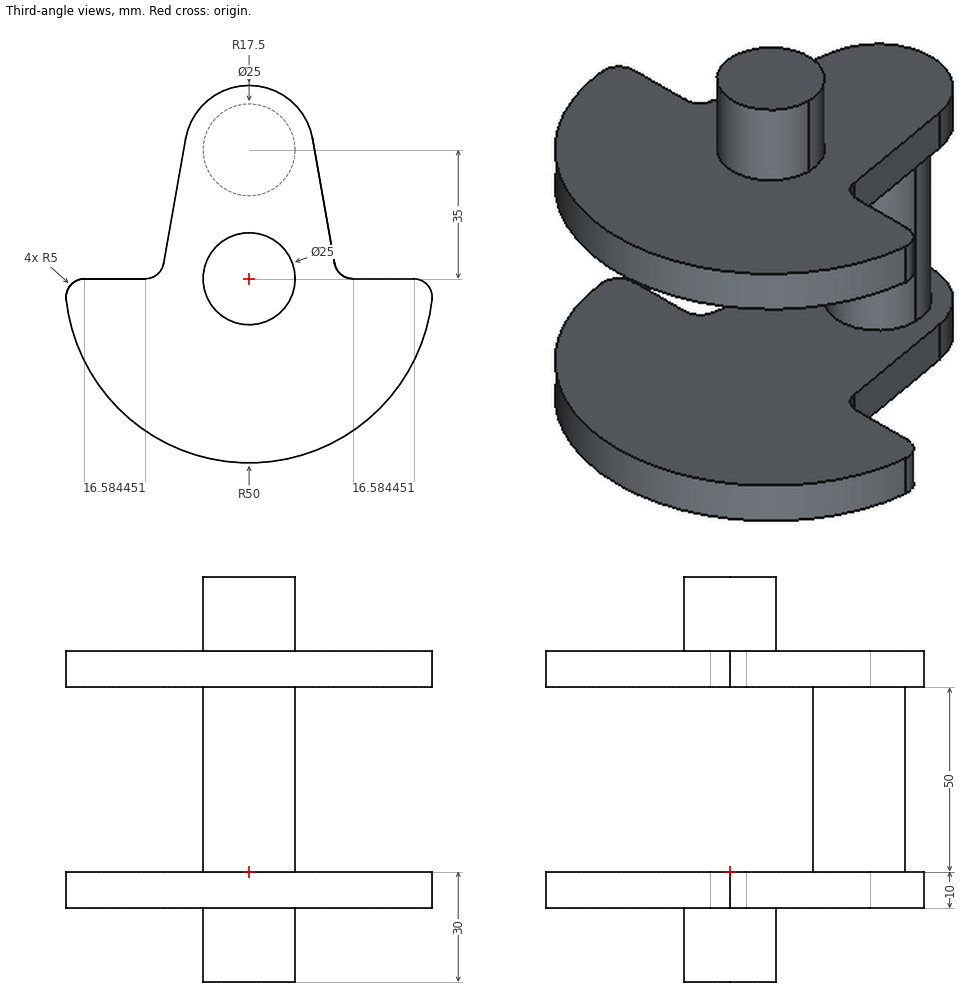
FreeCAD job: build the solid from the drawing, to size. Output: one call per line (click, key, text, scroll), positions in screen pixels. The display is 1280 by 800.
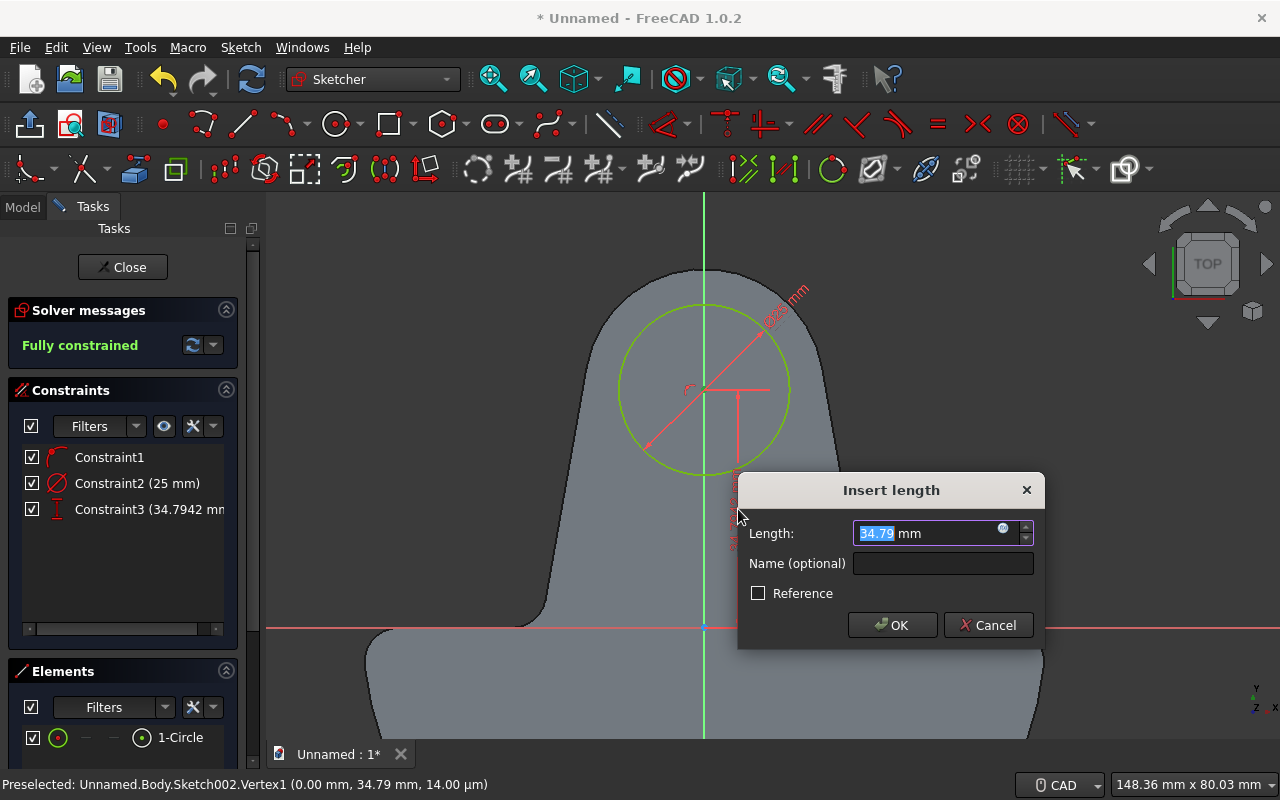
text(35)
key(Return)
key(Escape)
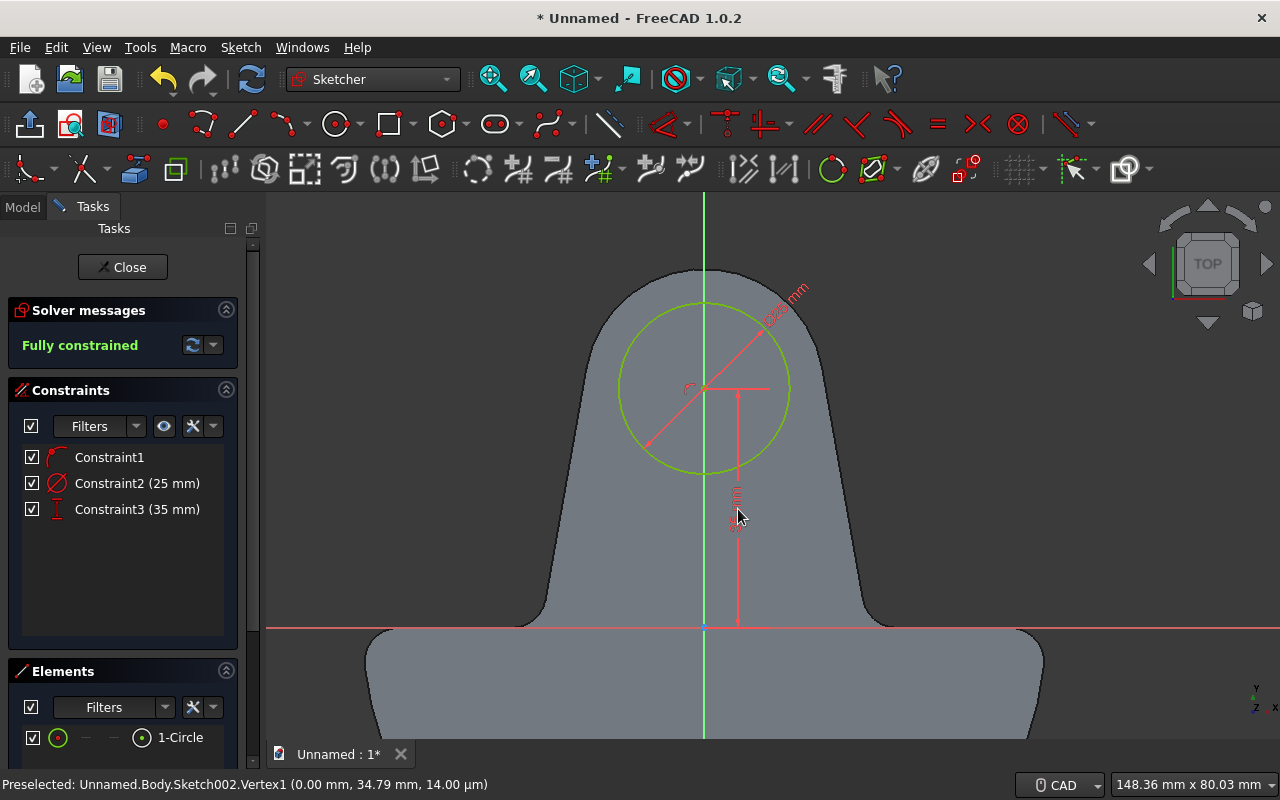
click(123, 267)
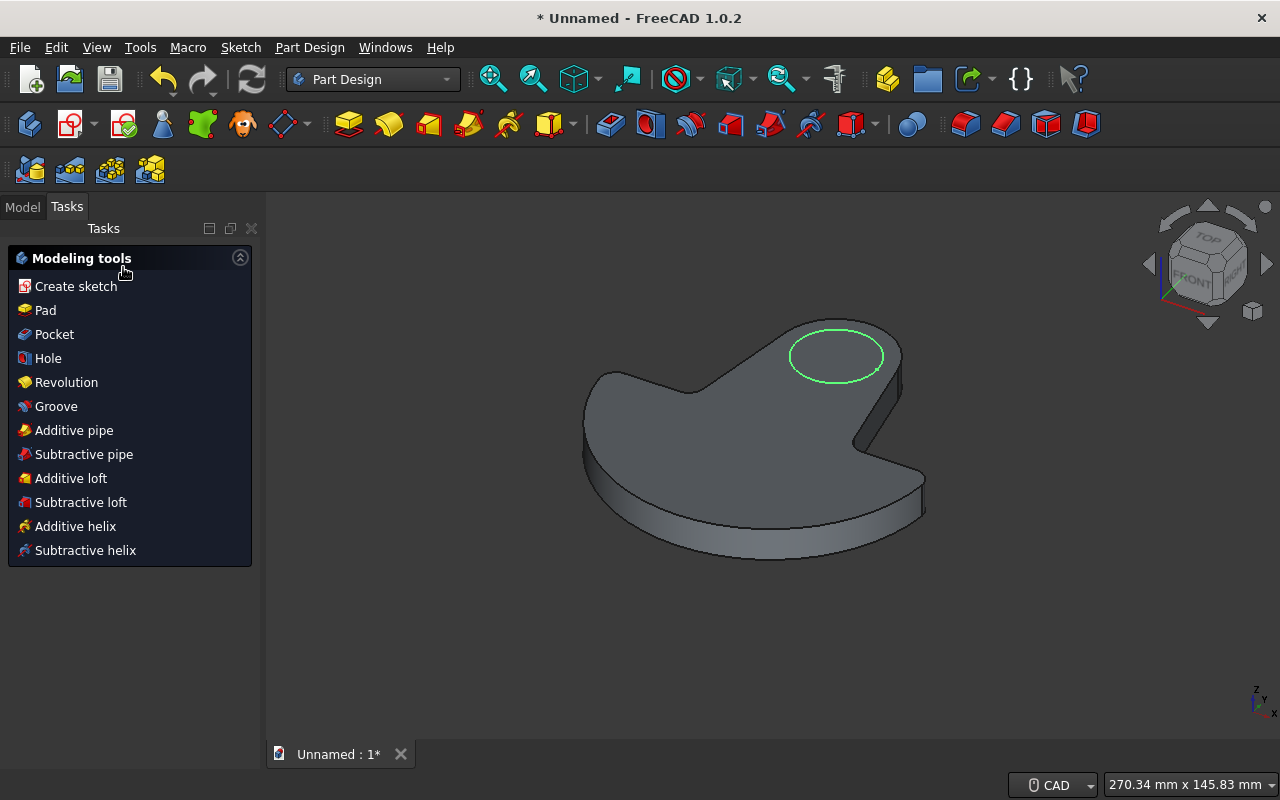
click(350, 124)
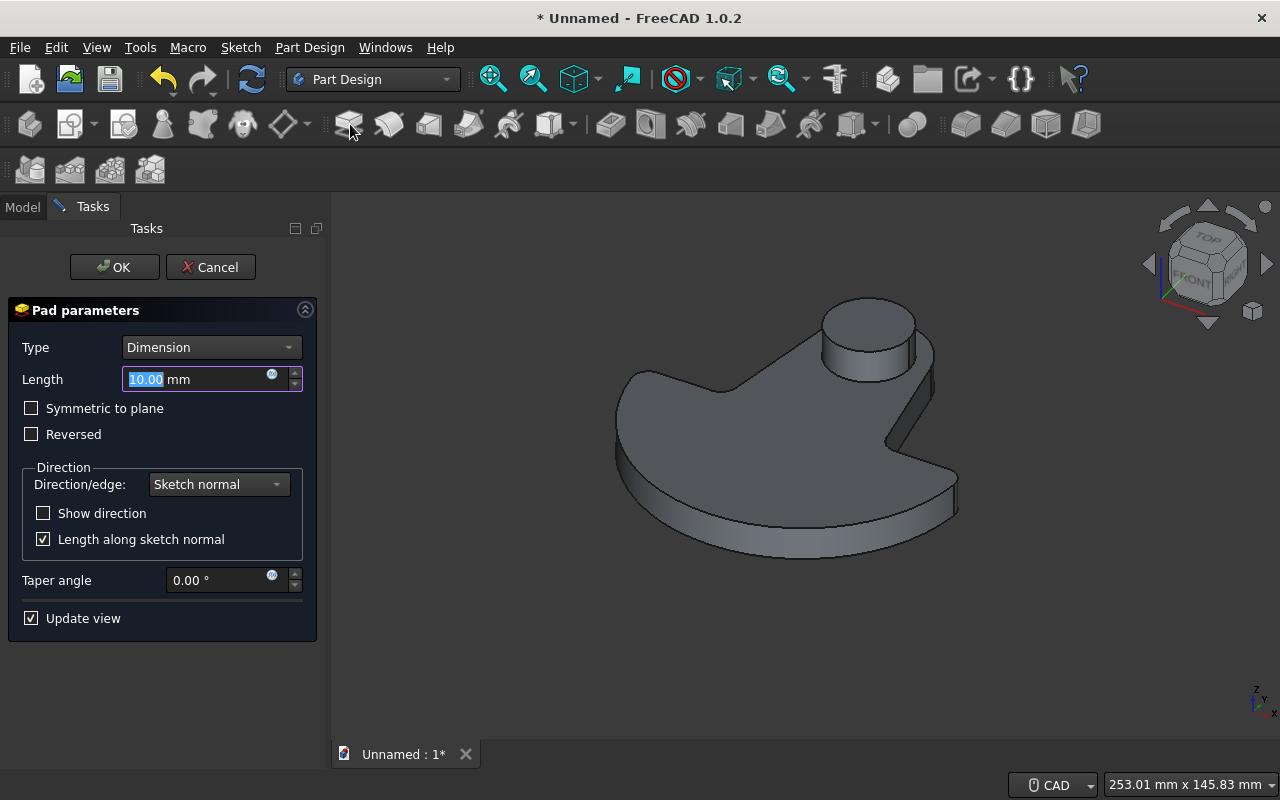
text(50)
key(Tab)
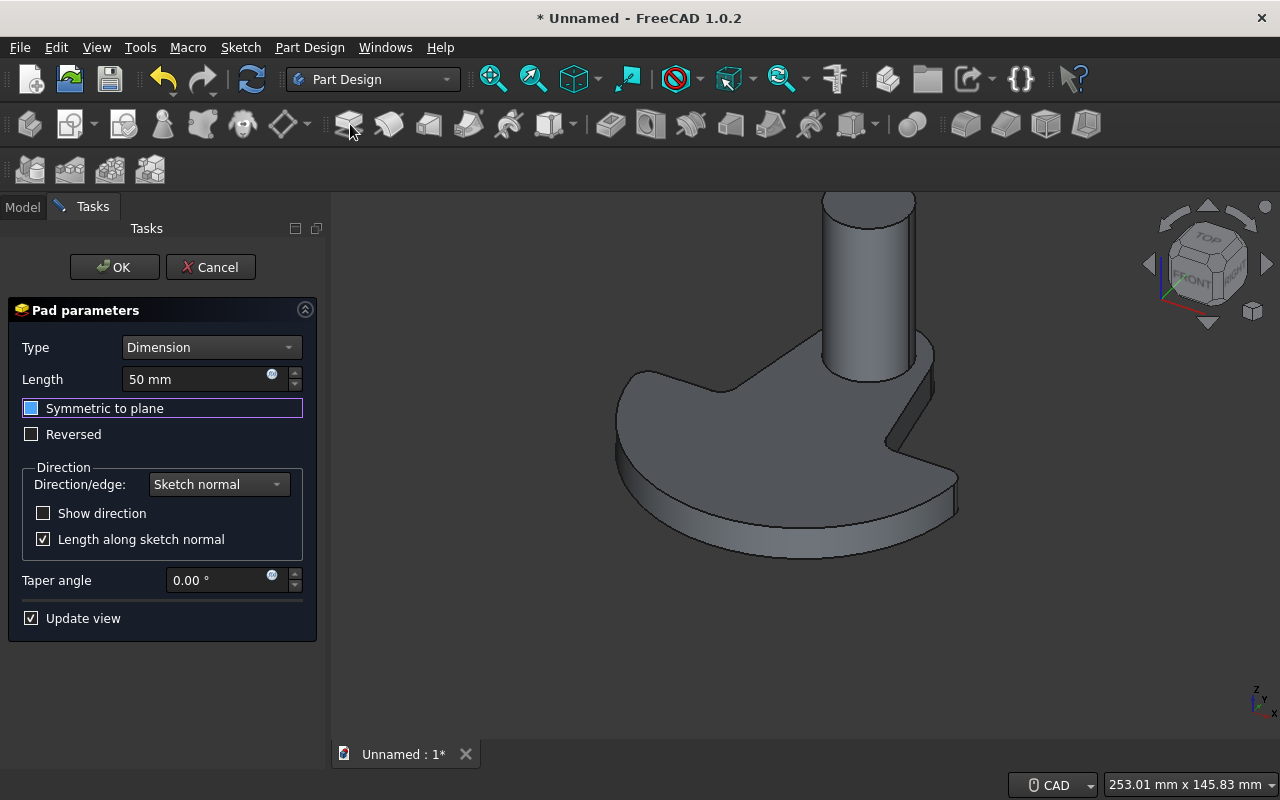
click(115, 267)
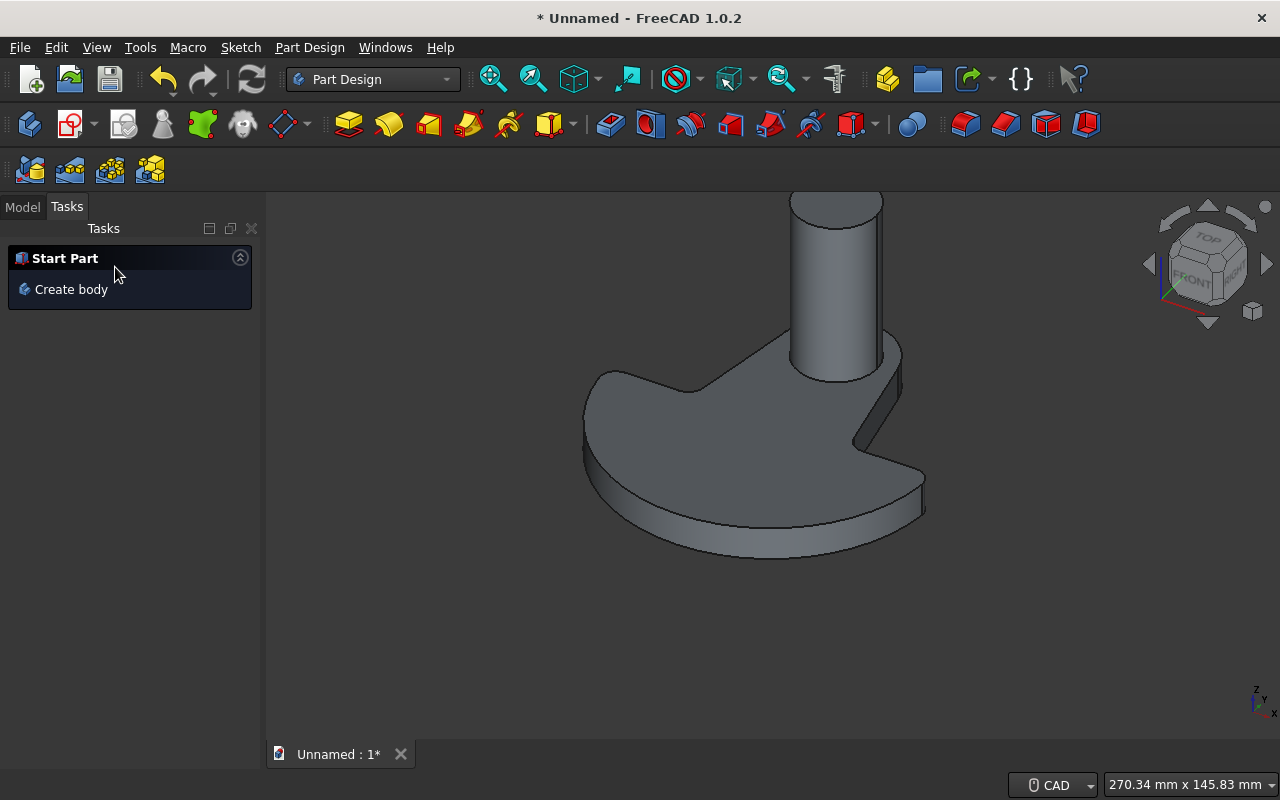
key(v)
key(f)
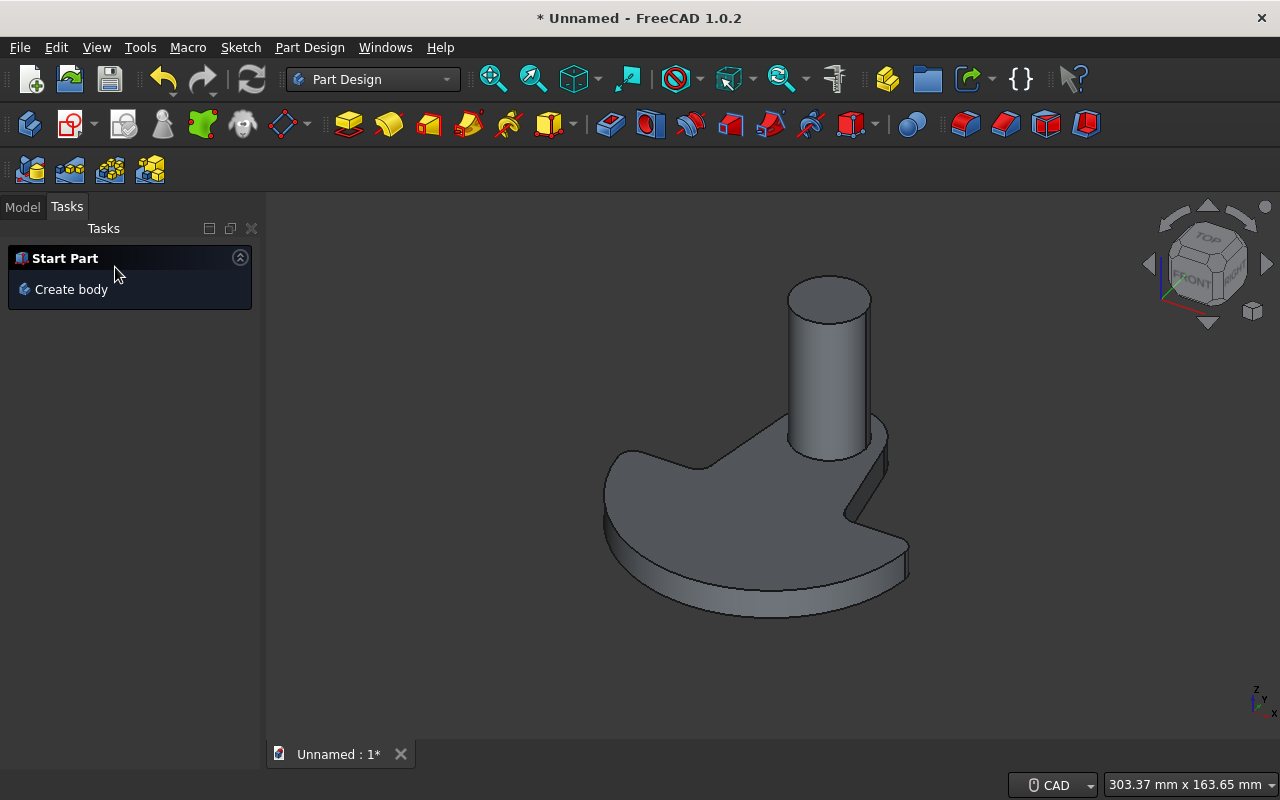
click(23, 206)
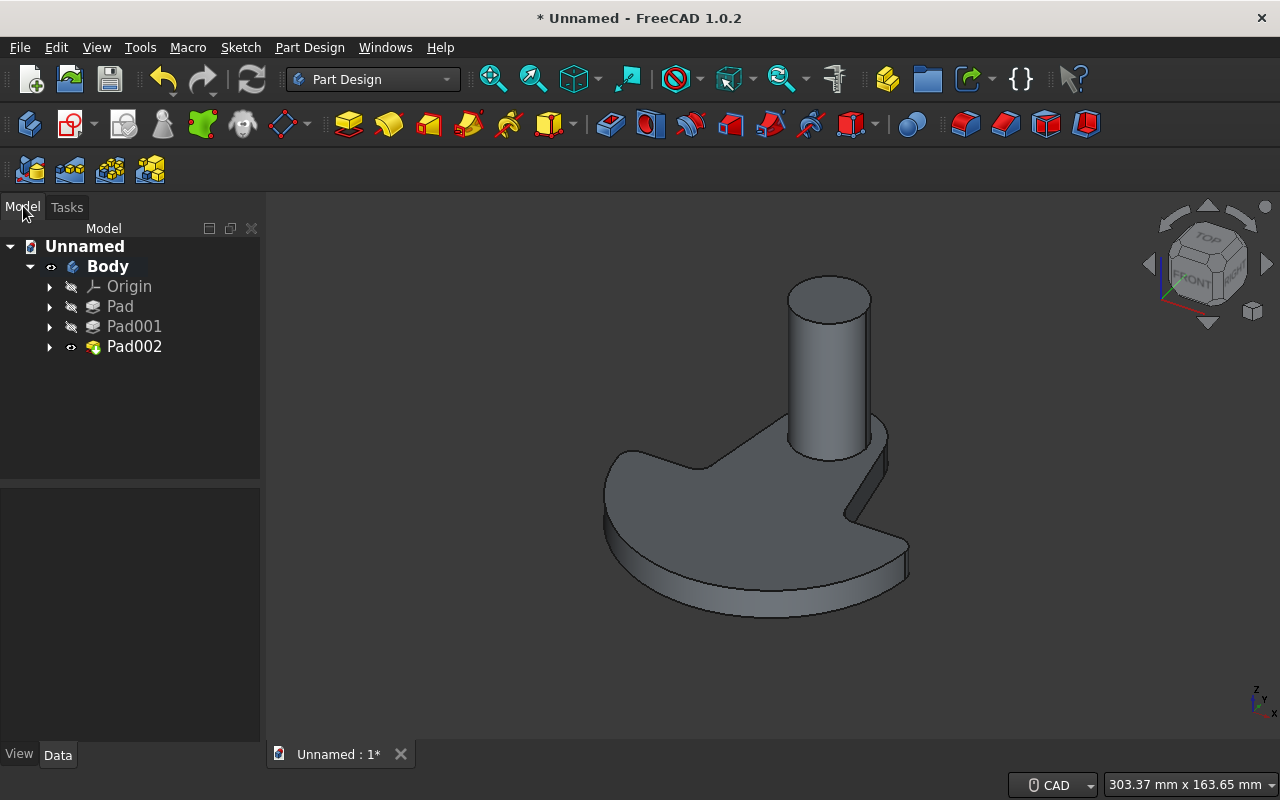
click(50, 287)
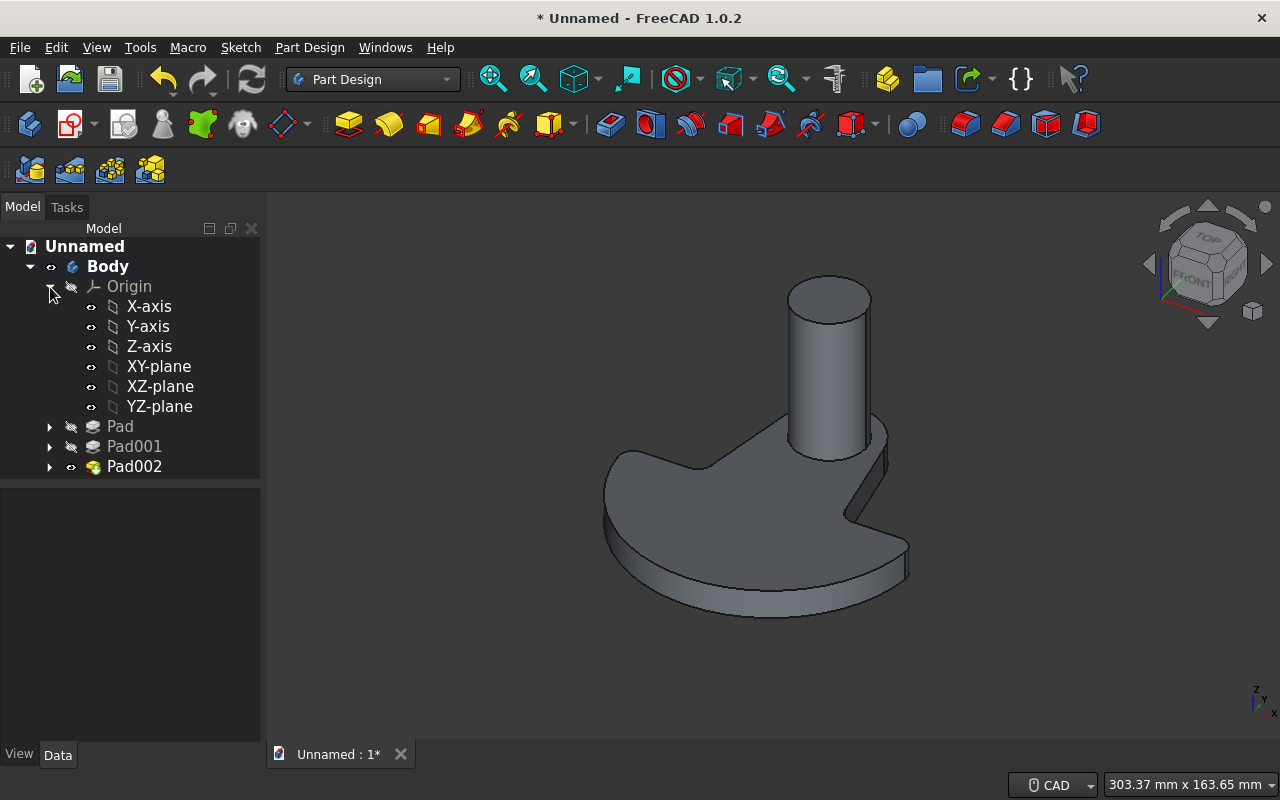
click(136, 367)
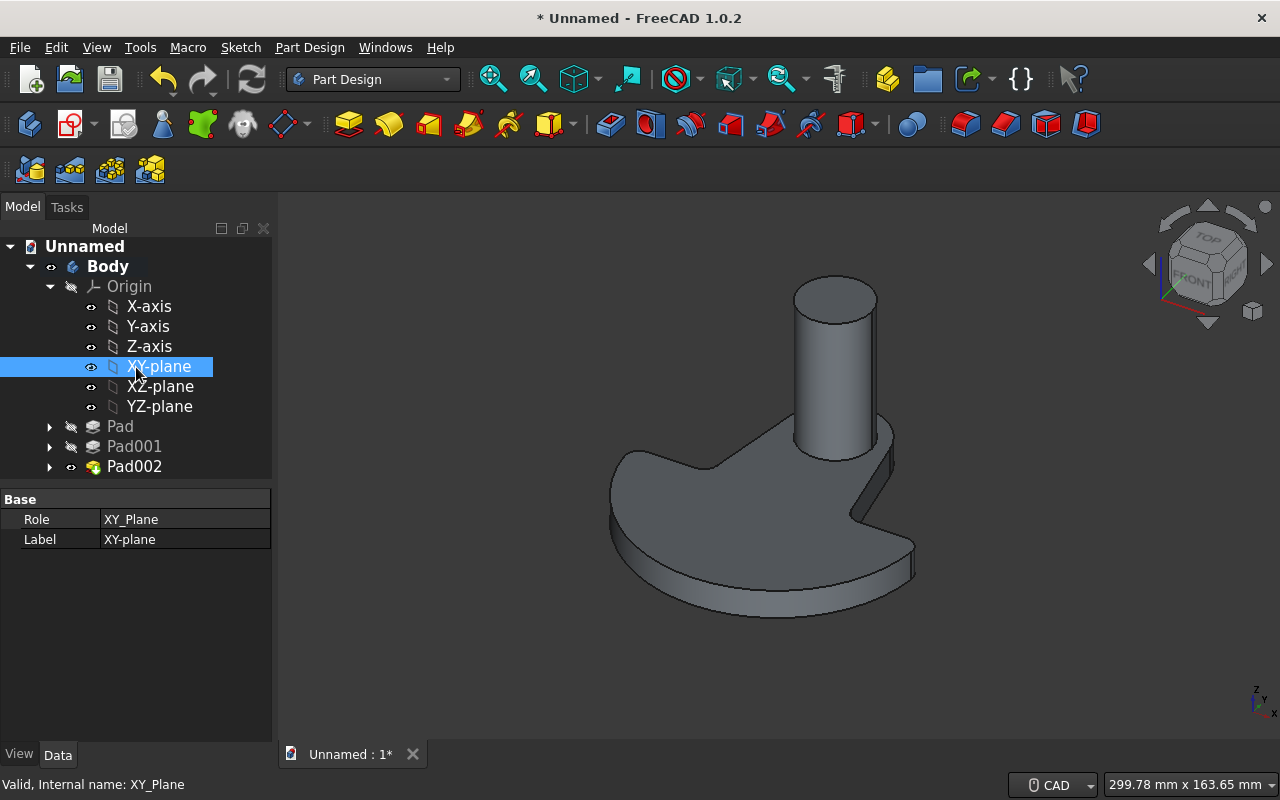
click(284, 124)